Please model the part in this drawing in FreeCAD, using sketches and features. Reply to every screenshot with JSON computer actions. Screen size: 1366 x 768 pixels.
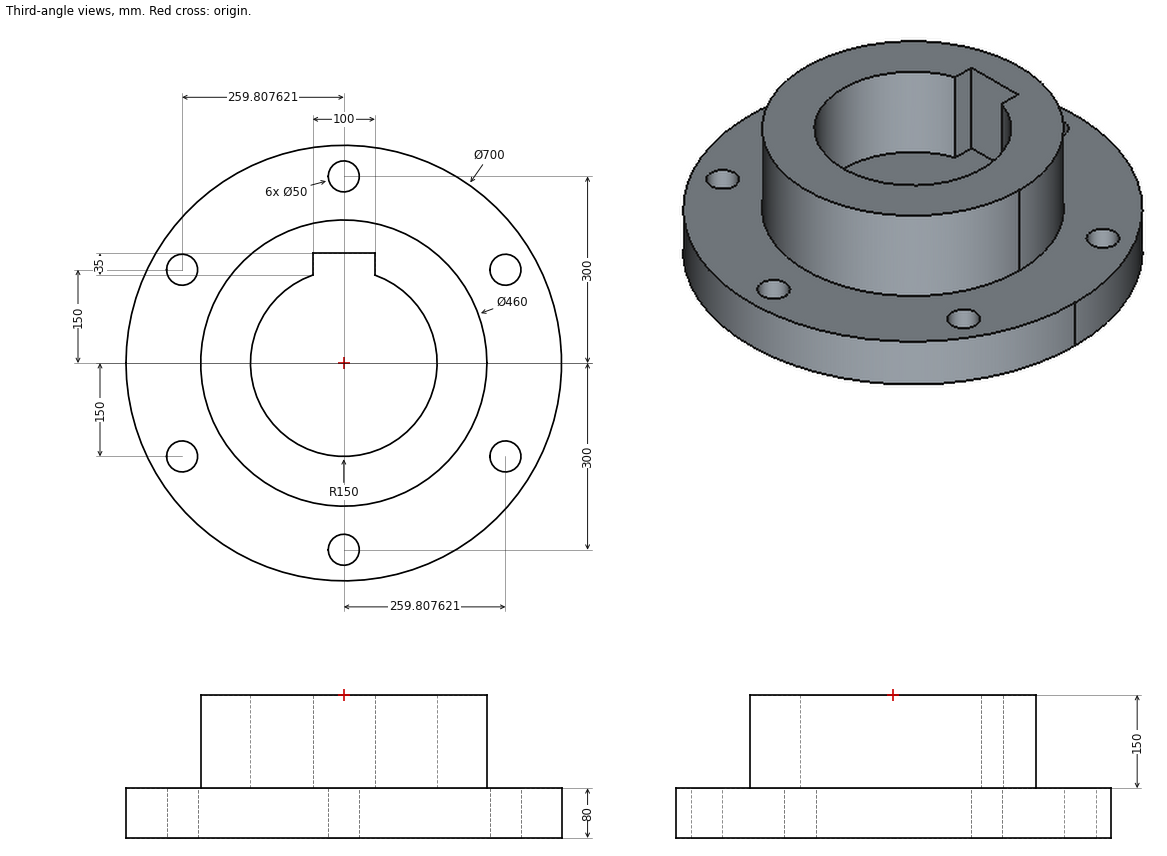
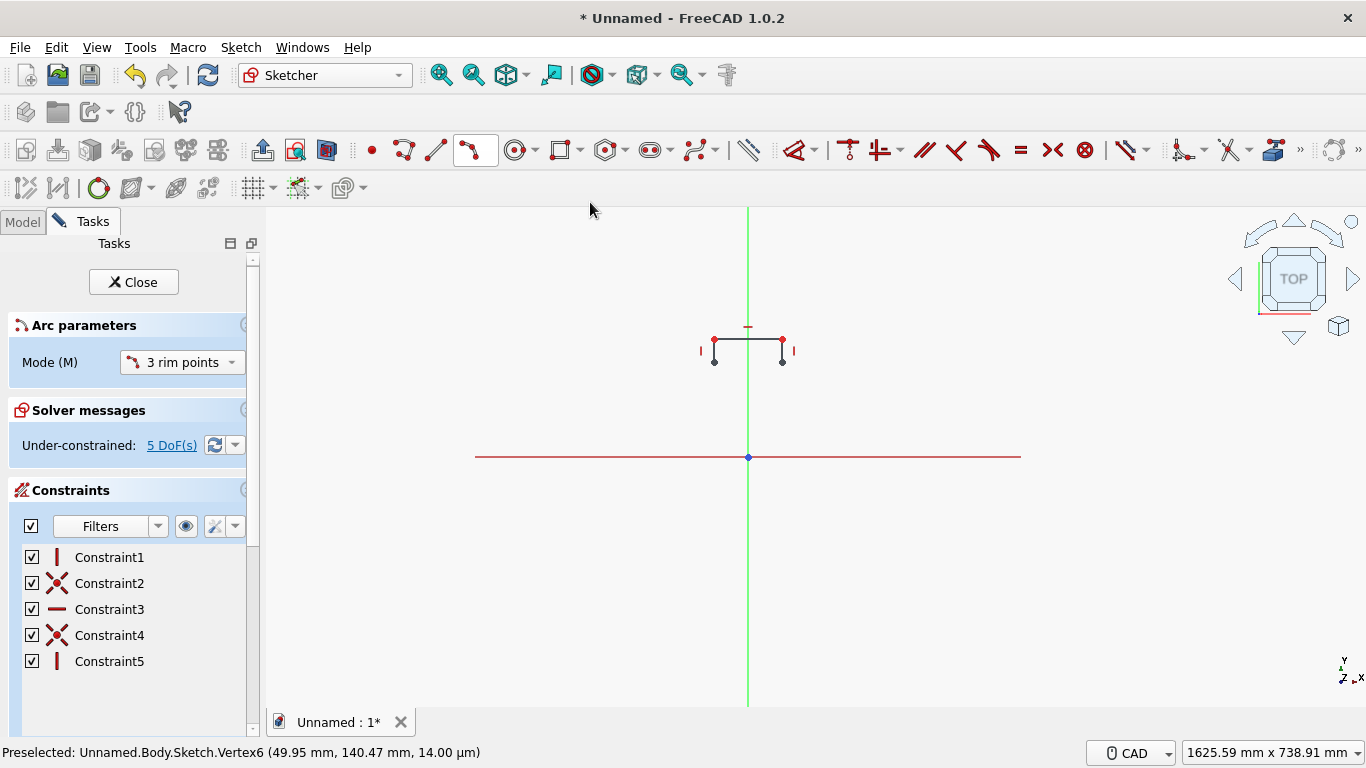
{"action": "scroll", "coordinate": [782, 362], "scroll_direction": "up", "scroll_amount": 2}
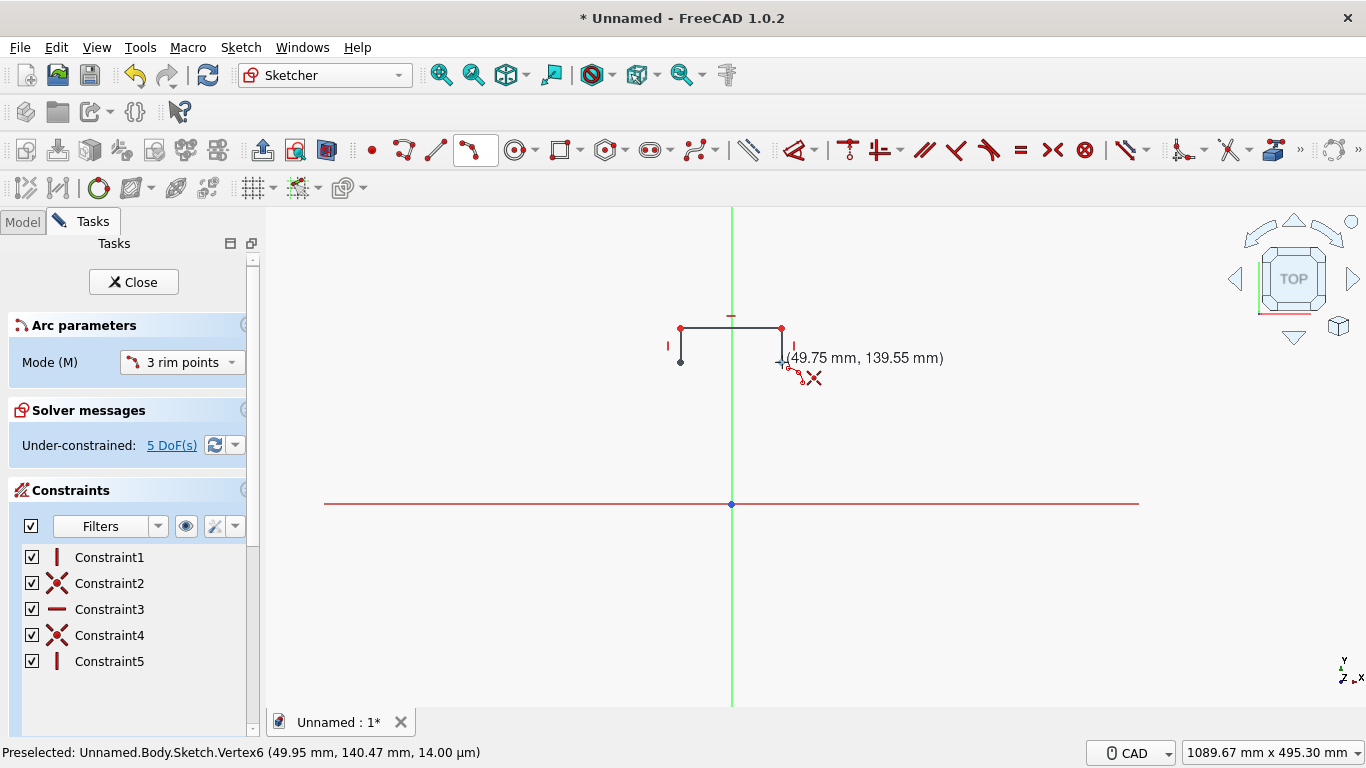
{"action": "left_click", "coordinate": [782, 362]}
{"action": "left_click", "coordinate": [681, 362]}
{"action": "left_click", "coordinate": [651, 632]}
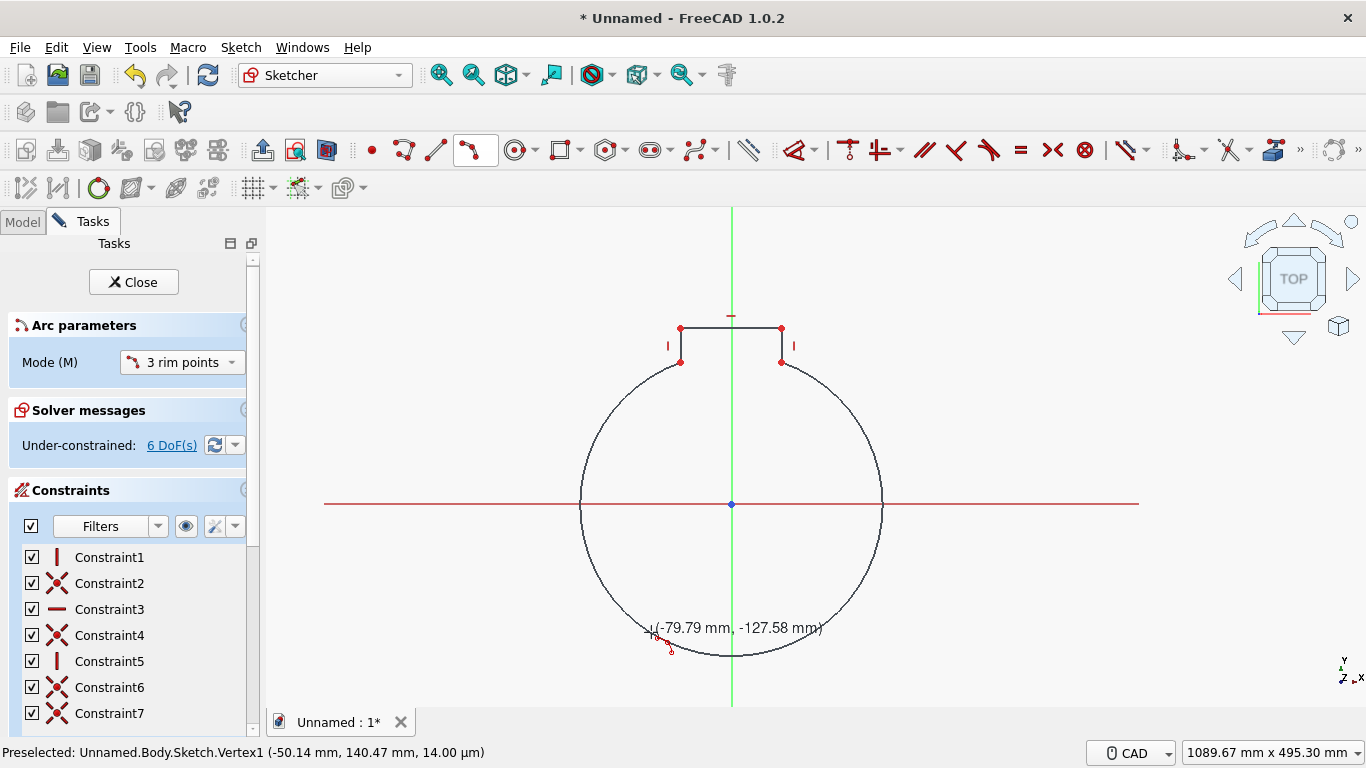
{"action": "left_click", "coordinate": [516, 150]}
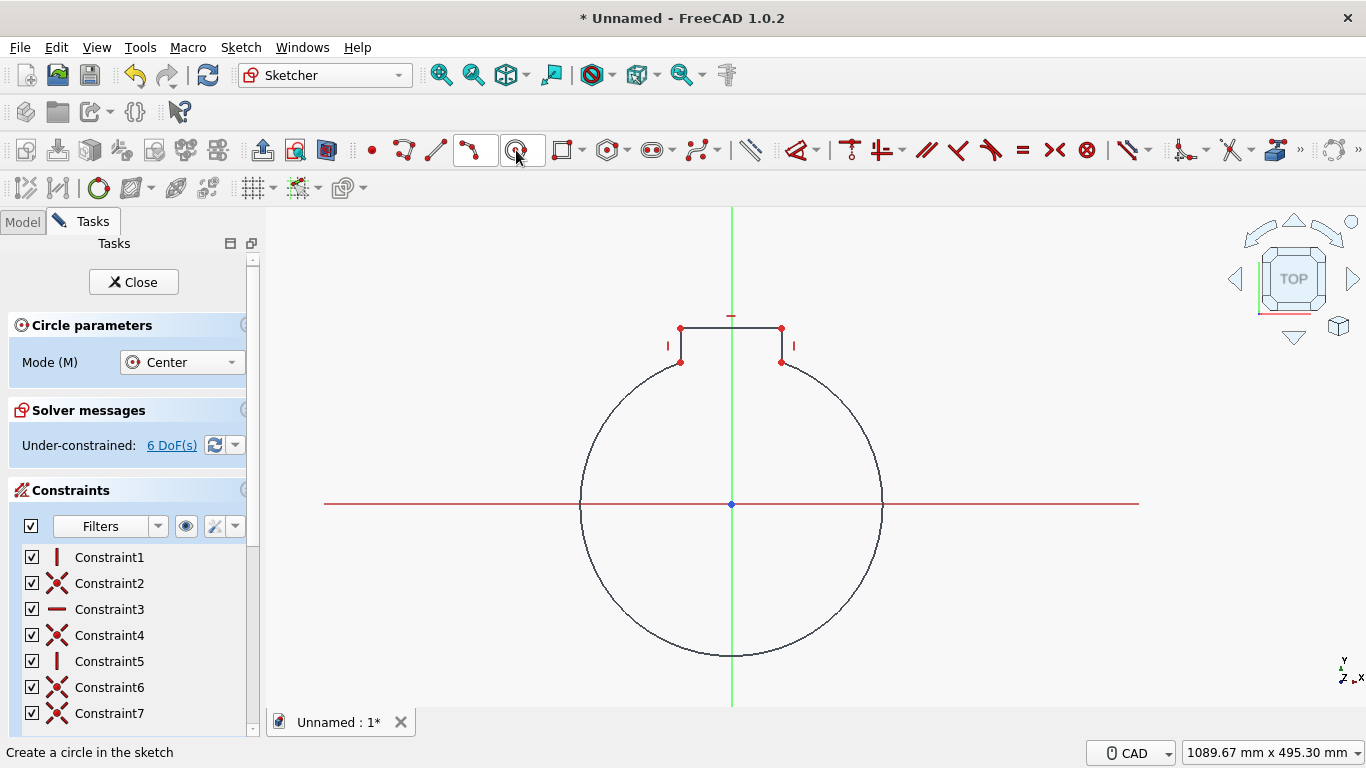
{"action": "left_click", "coordinate": [732, 504]}
{"action": "mouse_move", "coordinate": [896, 340]}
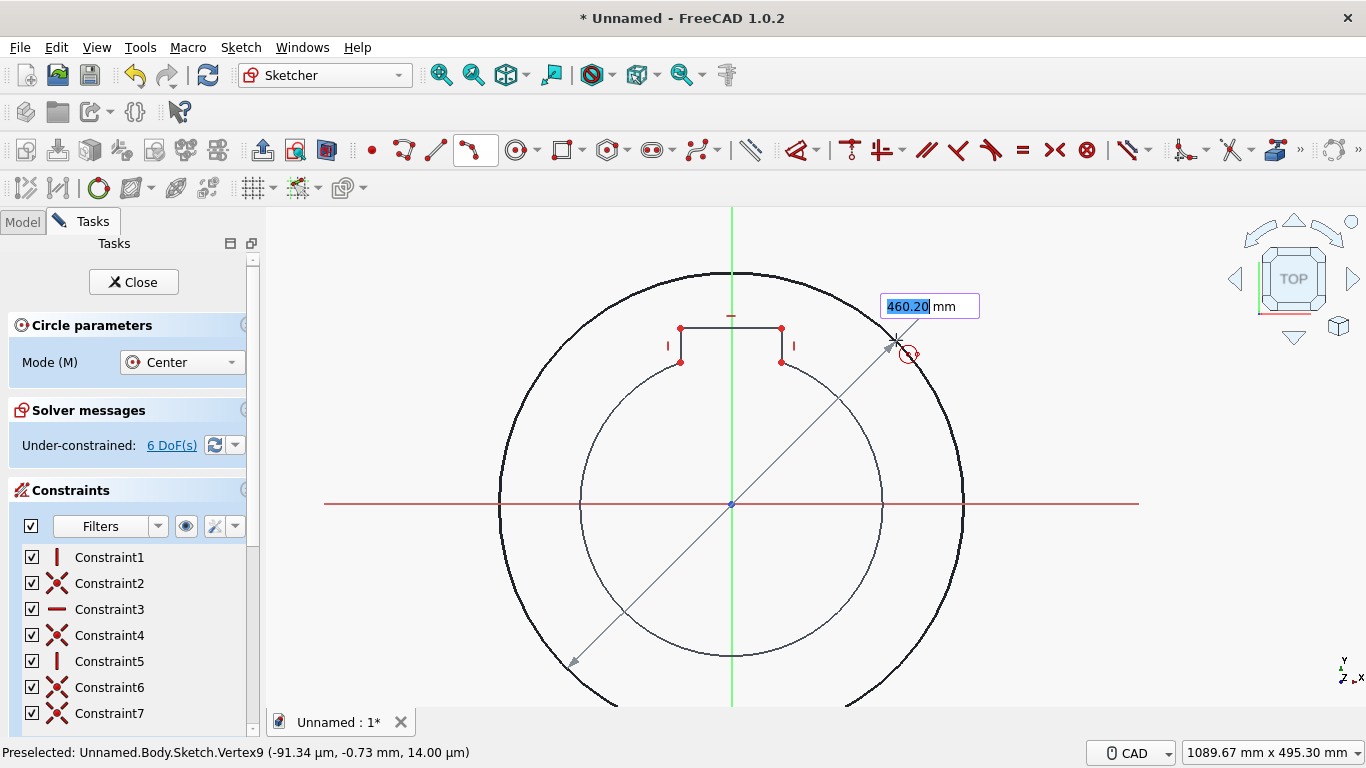
{"action": "type", "text": "460"}
{"action": "key", "text": "Return"}
{"action": "key", "text": "Escape"}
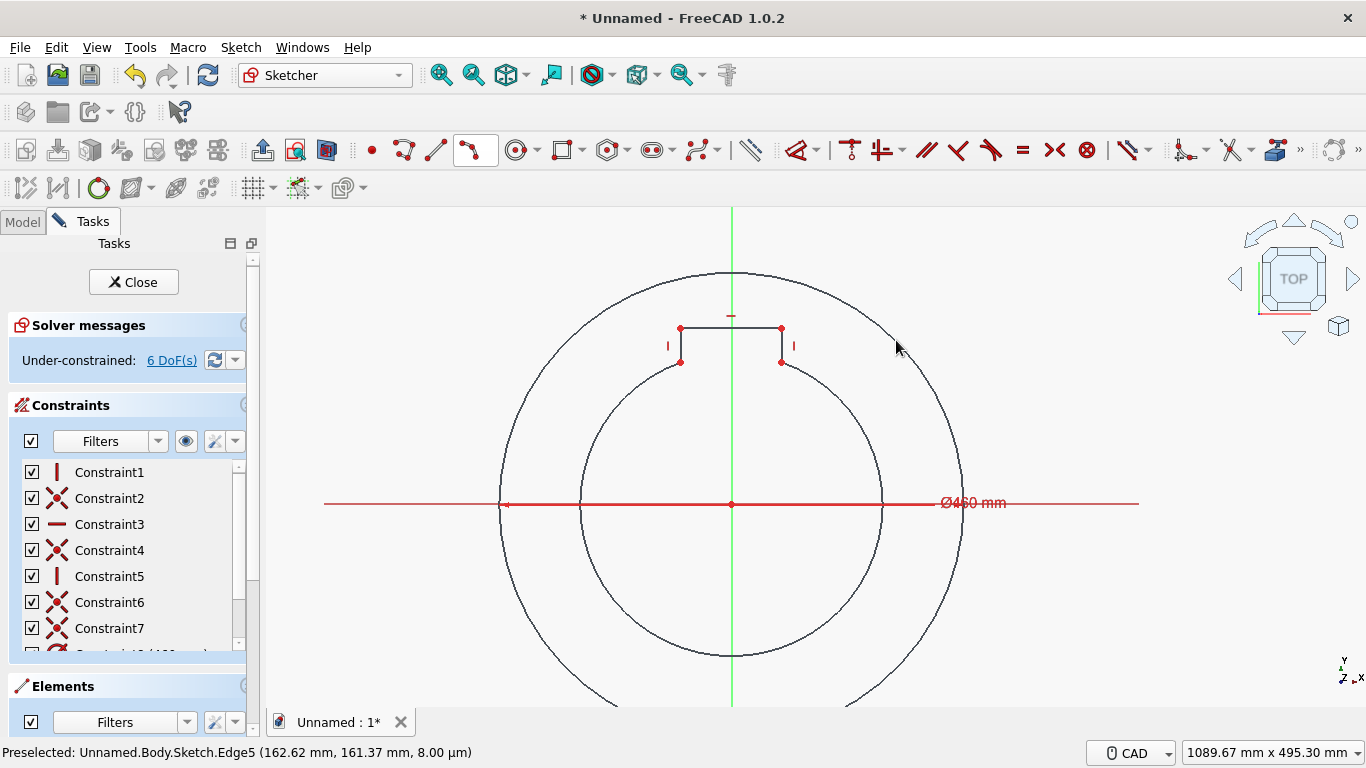
{"action": "left_click_drag", "start_coordinate": [721, 494], "coordinate": [742, 515]}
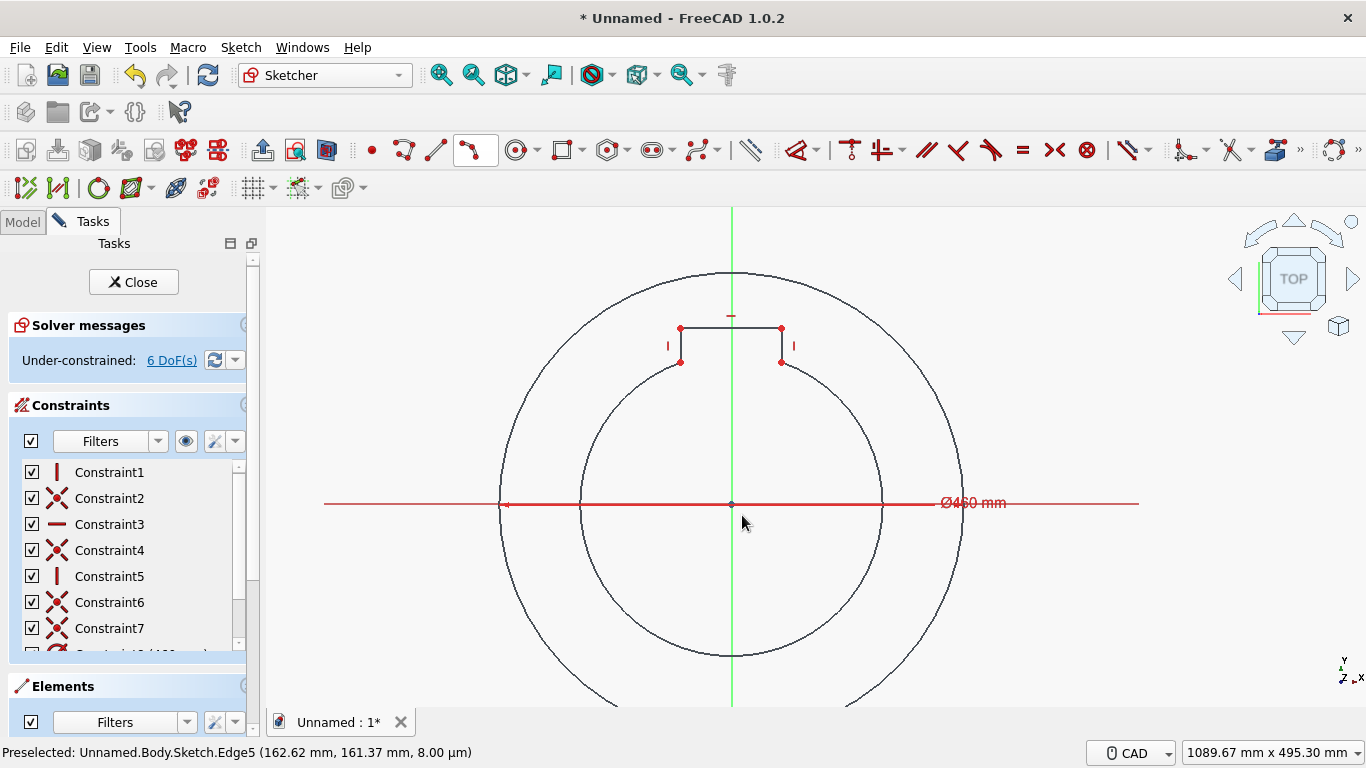
{"action": "left_click", "coordinate": [850, 150]}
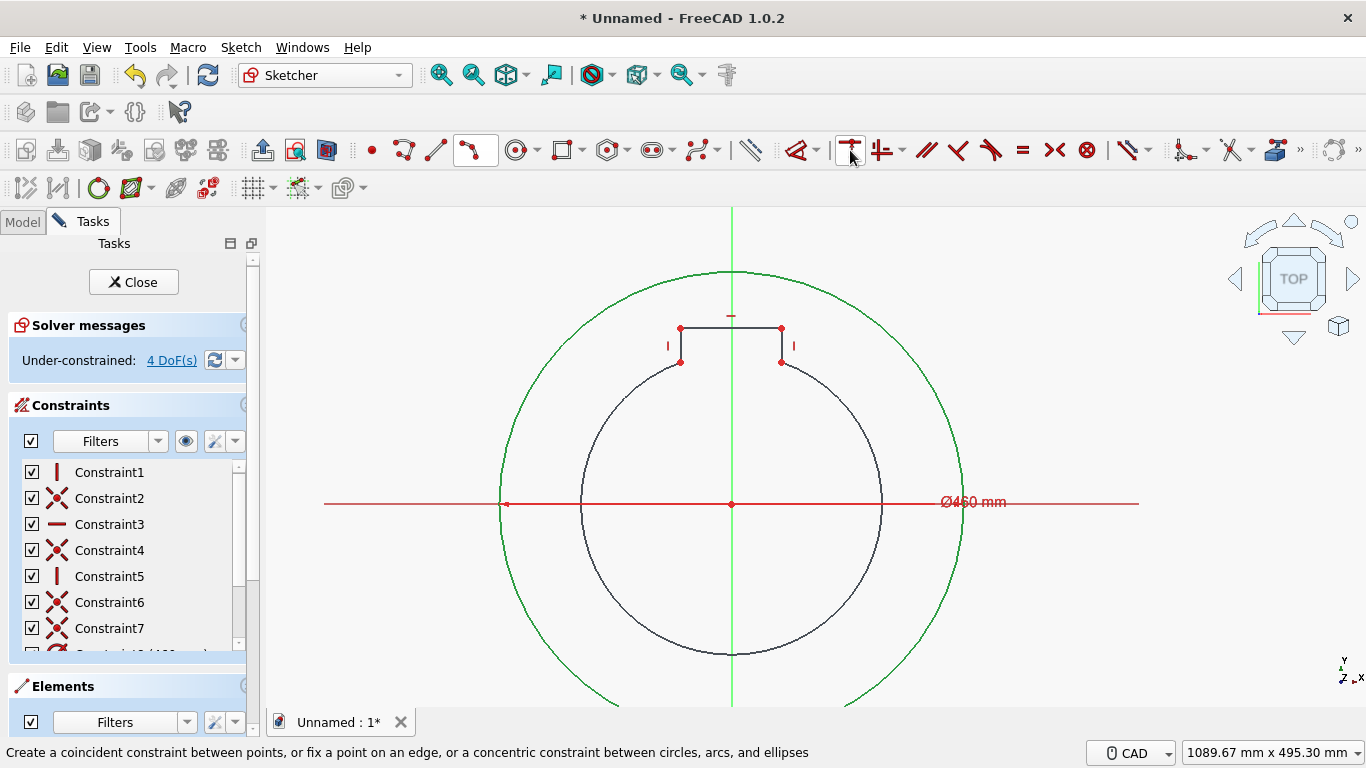
{"action": "key", "text": "d"}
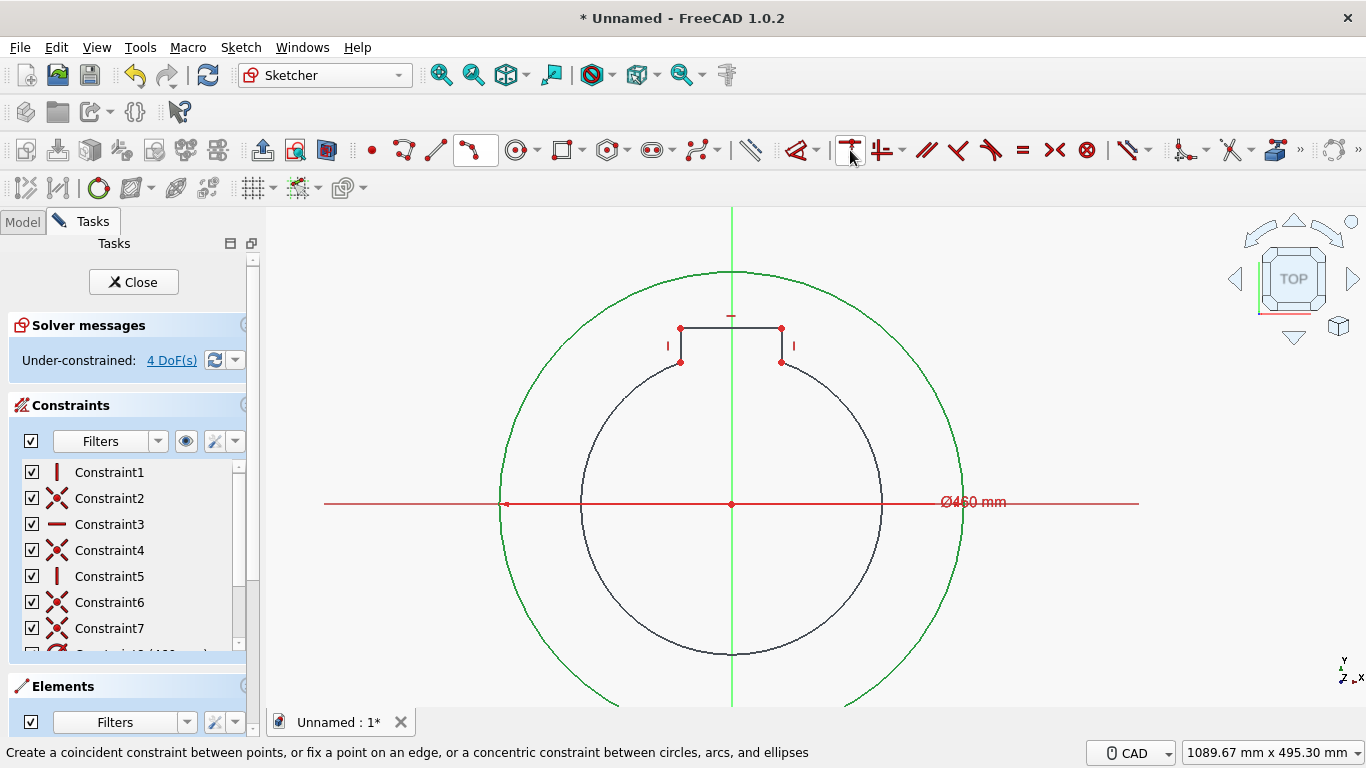
{"action": "left_click", "coordinate": [596, 570]}
{"action": "left_click", "coordinate": [567, 584]}